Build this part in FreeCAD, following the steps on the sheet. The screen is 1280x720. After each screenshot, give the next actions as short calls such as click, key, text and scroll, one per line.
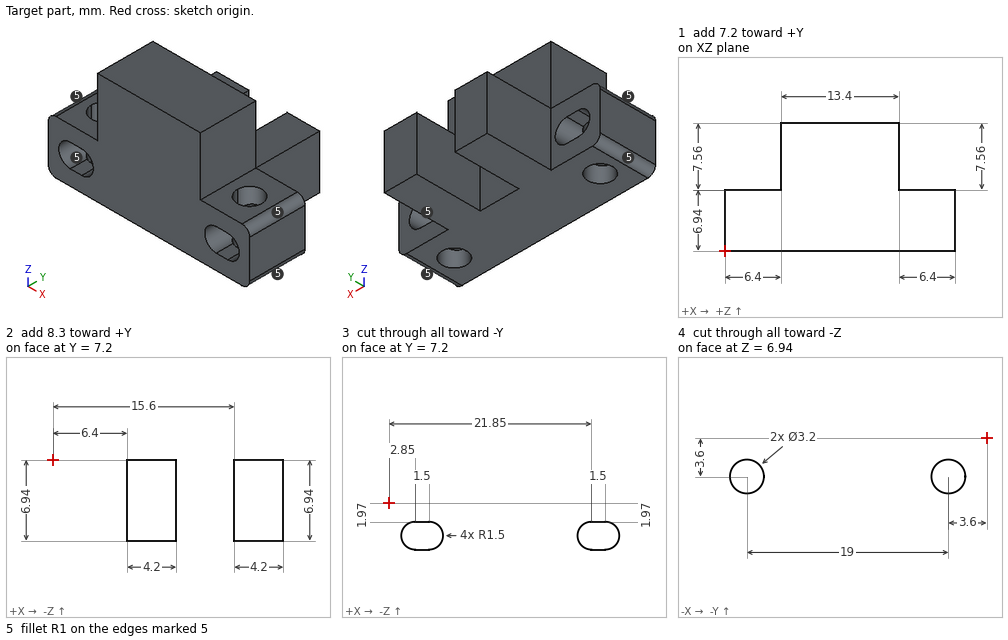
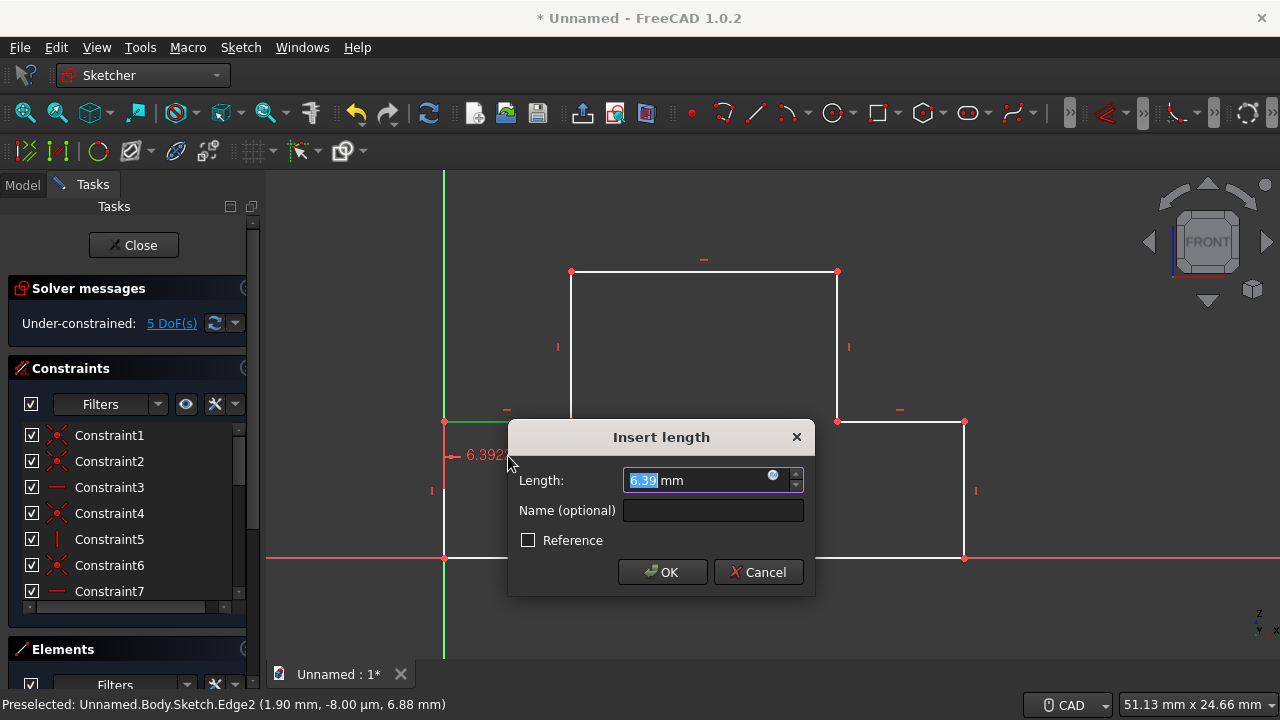
text(6.4)
key(Return)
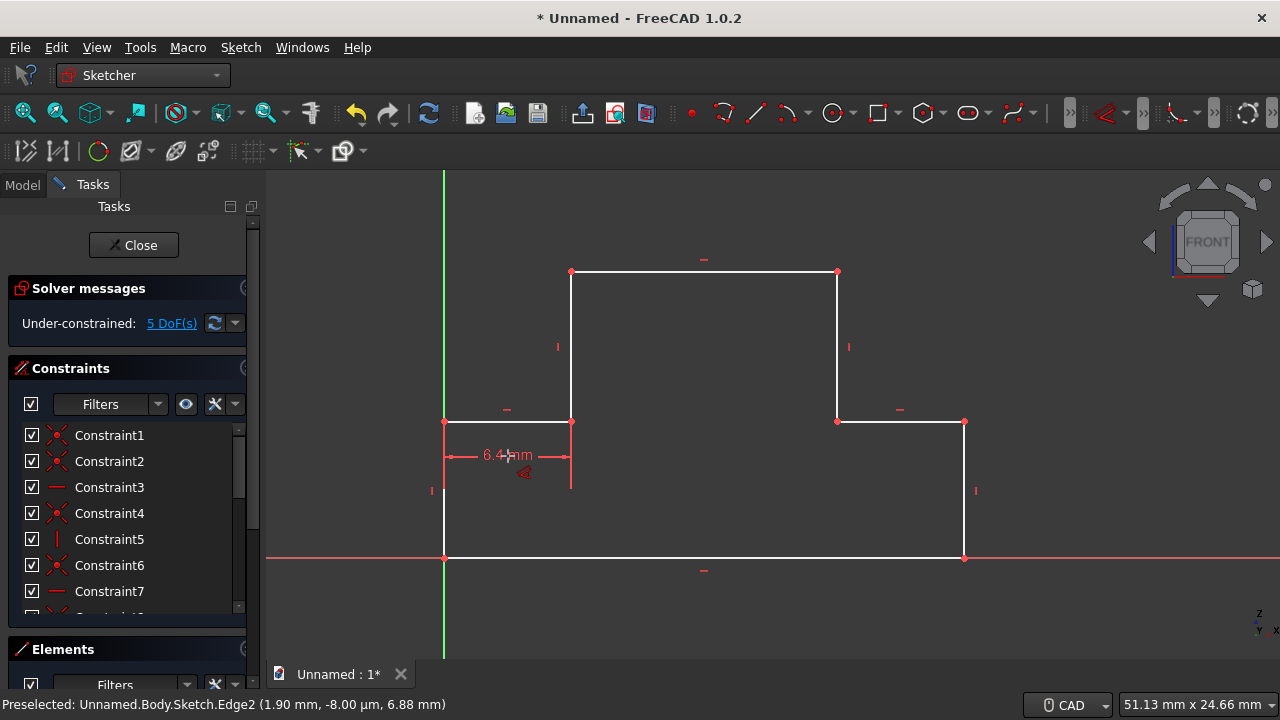
click(875, 422)
click(900, 456)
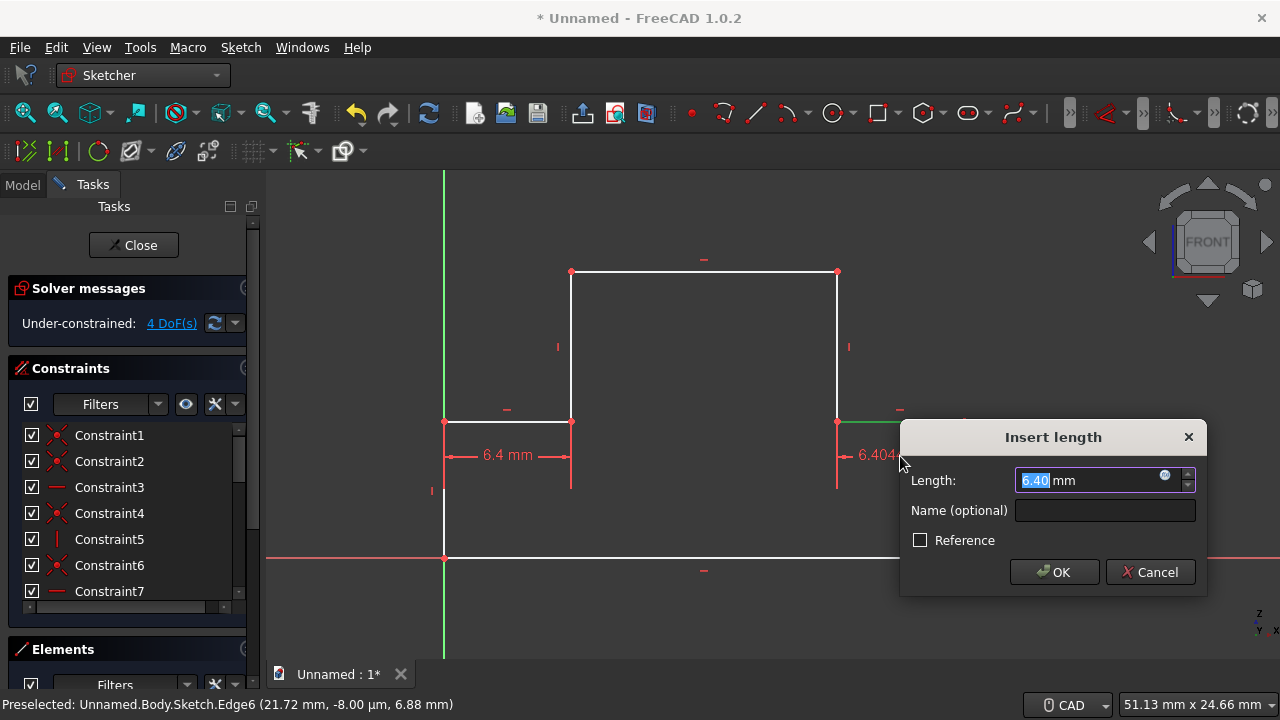
text(6.4)
key(Return)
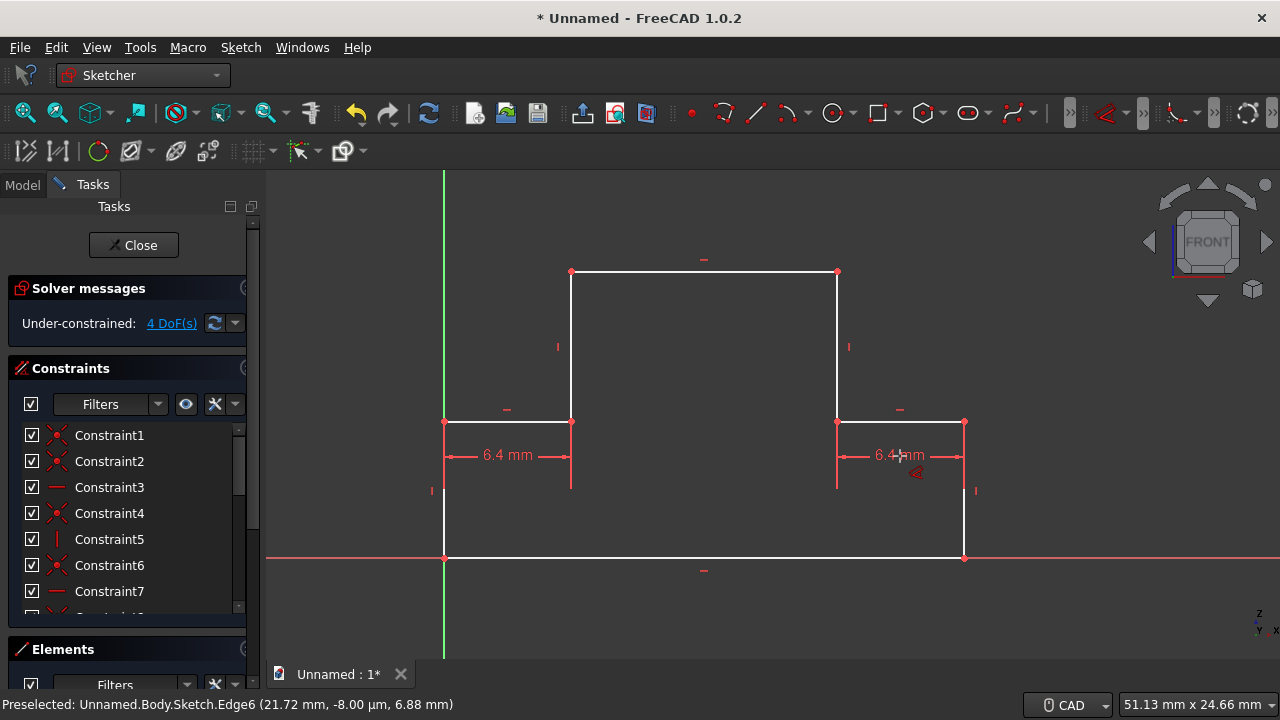
click(444, 517)
click(410, 490)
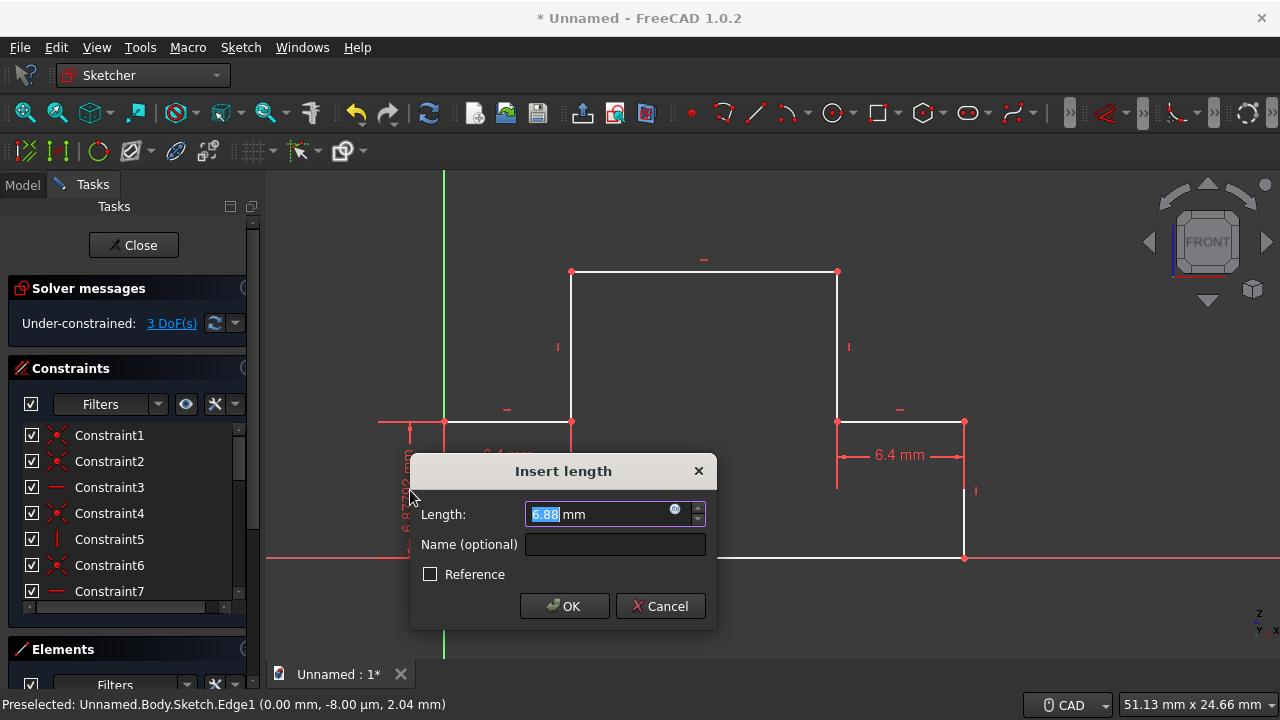
text(6.94)
key(Return)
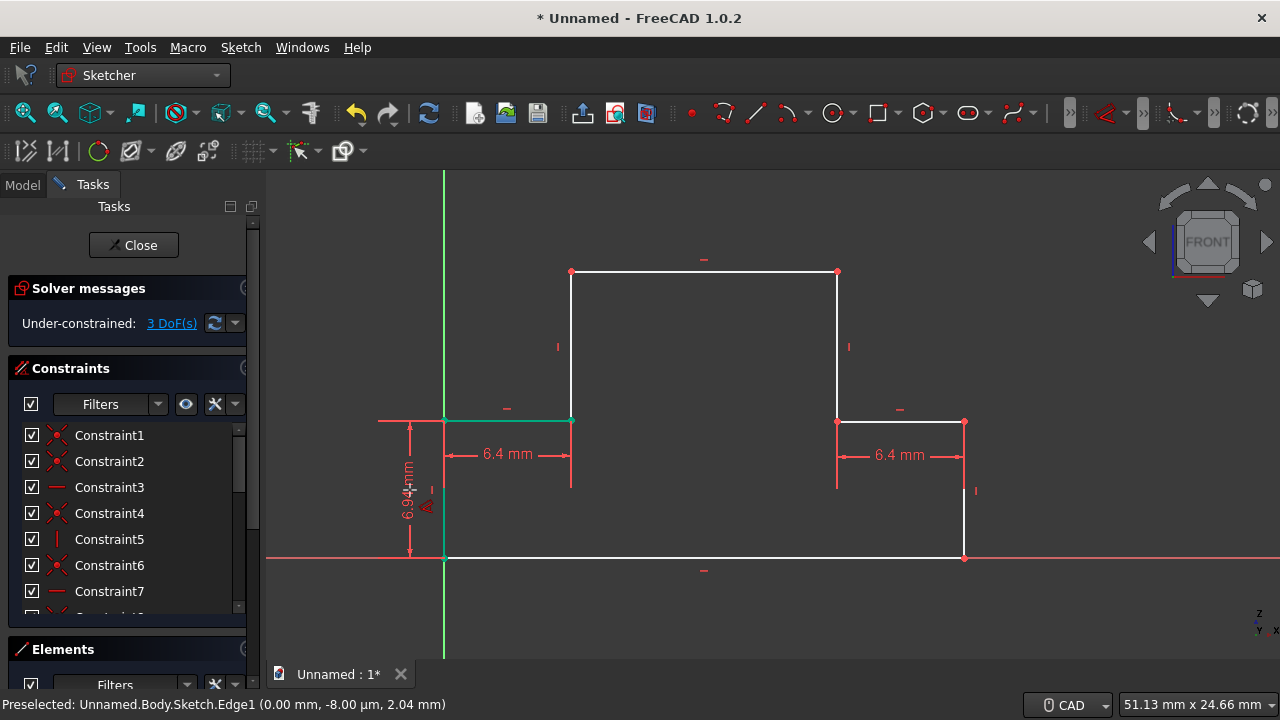
click(571, 376)
click(537, 346)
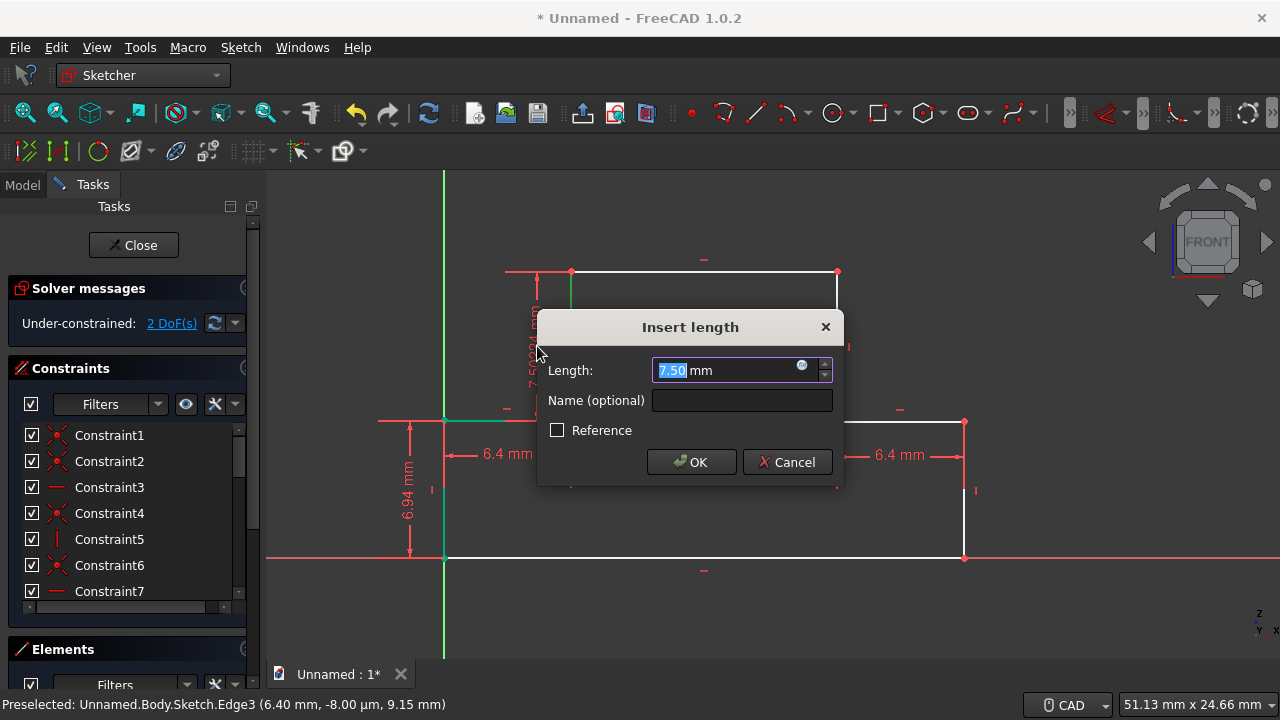
text(7.56)
key(Return)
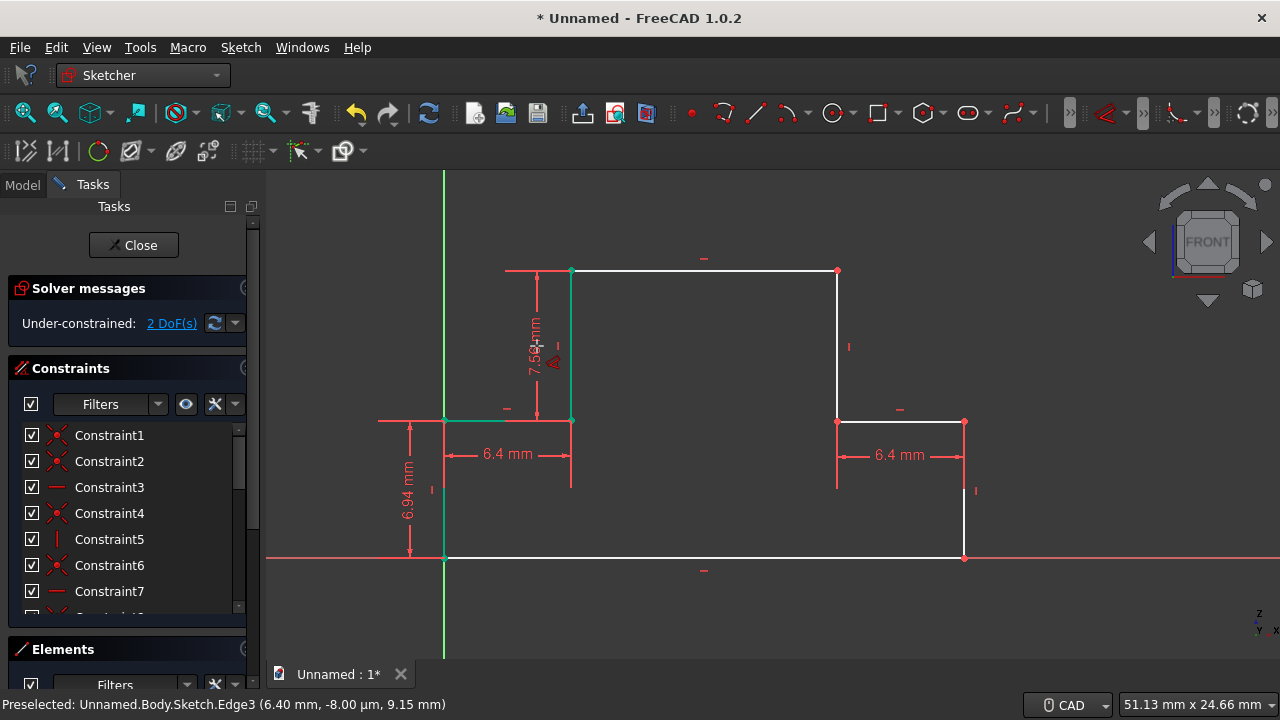
click(651, 271)
click(704, 237)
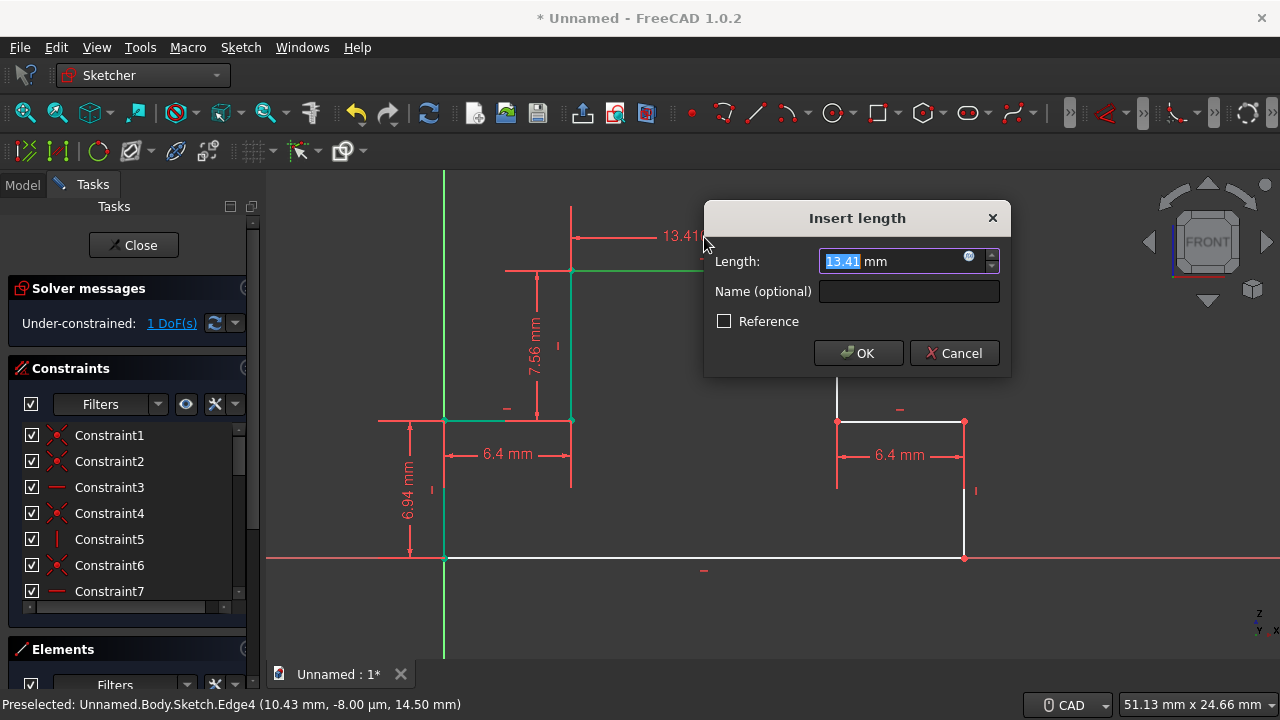
text(13.4)
key(Return)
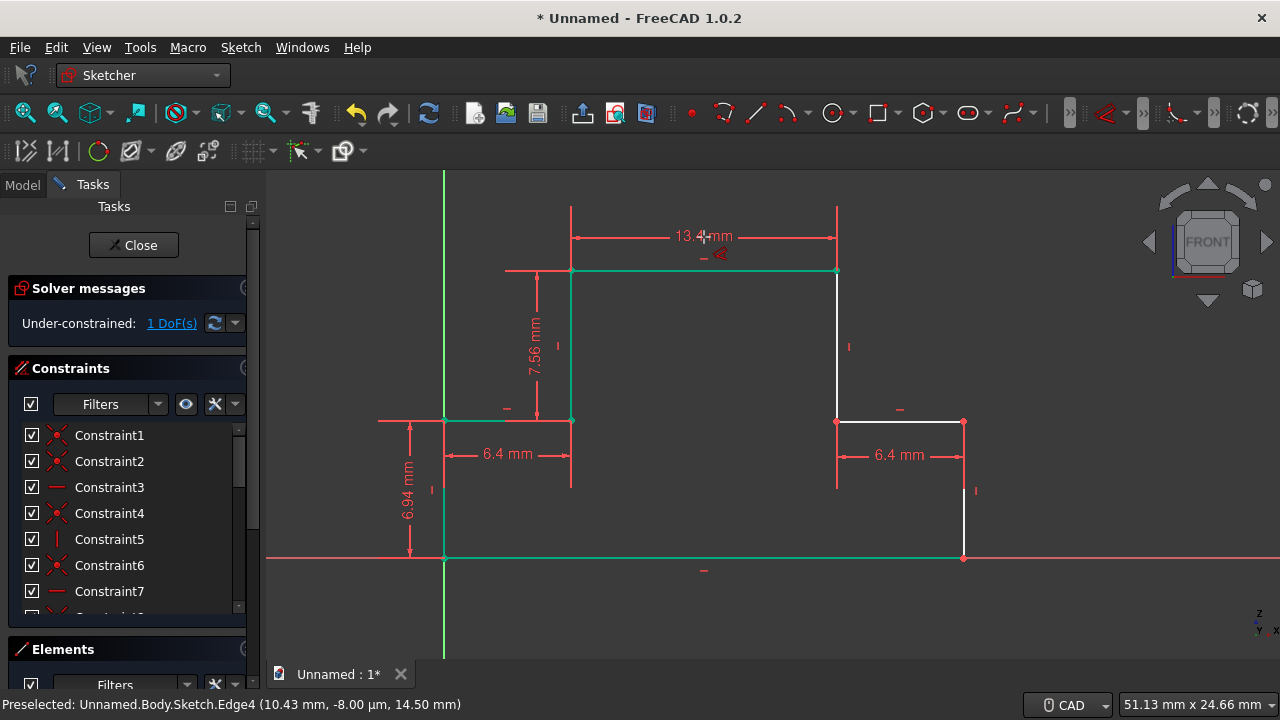
click(837, 316)
click(871, 346)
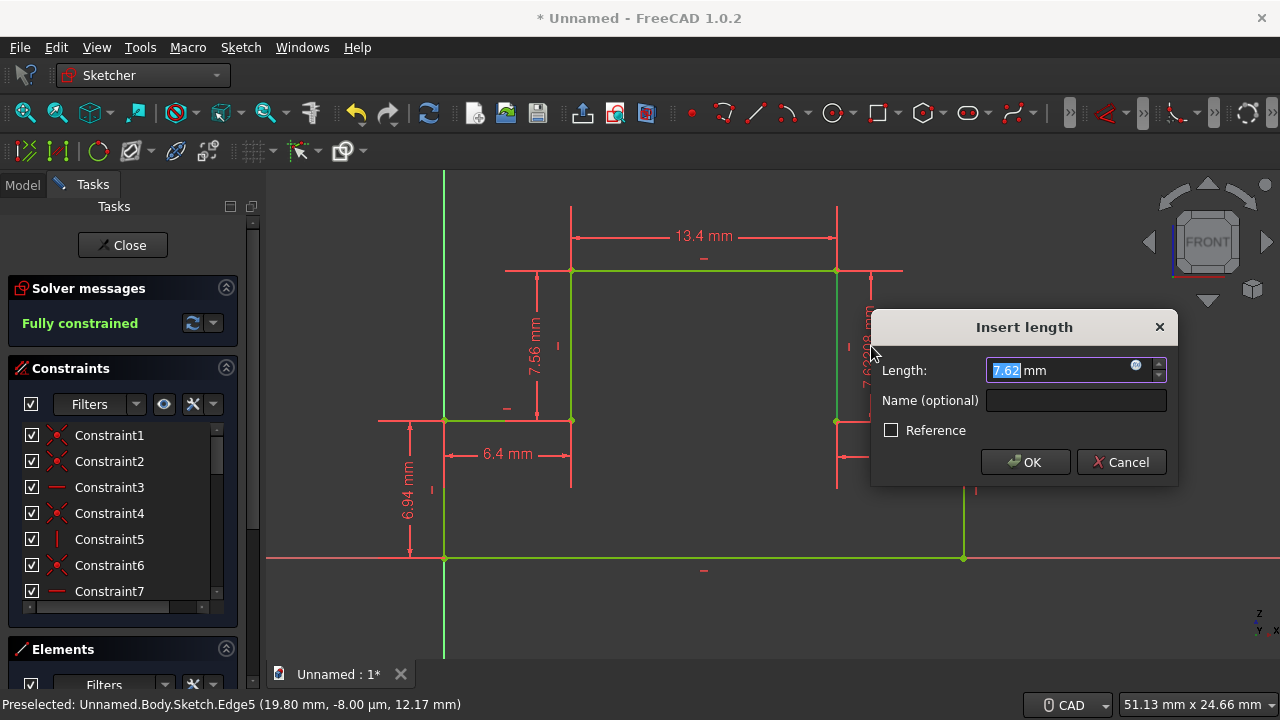
text(7.56)
key(Return)
key(Escape)